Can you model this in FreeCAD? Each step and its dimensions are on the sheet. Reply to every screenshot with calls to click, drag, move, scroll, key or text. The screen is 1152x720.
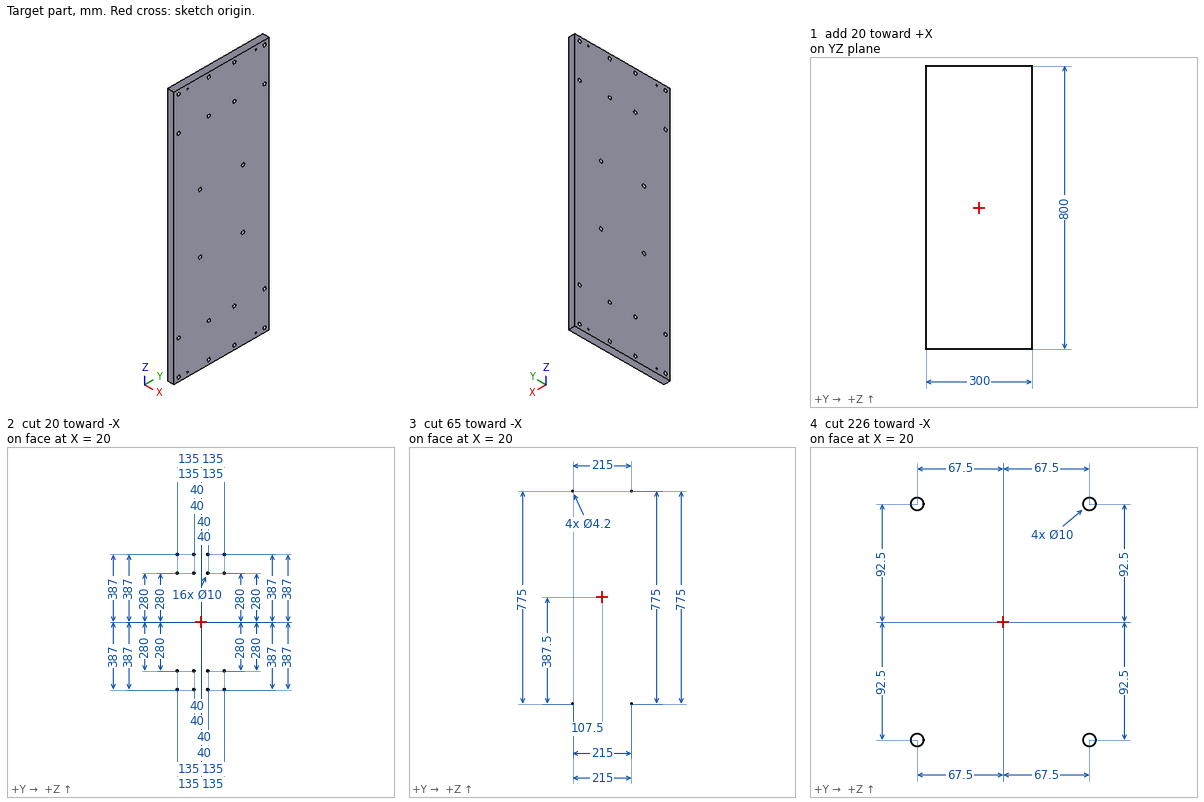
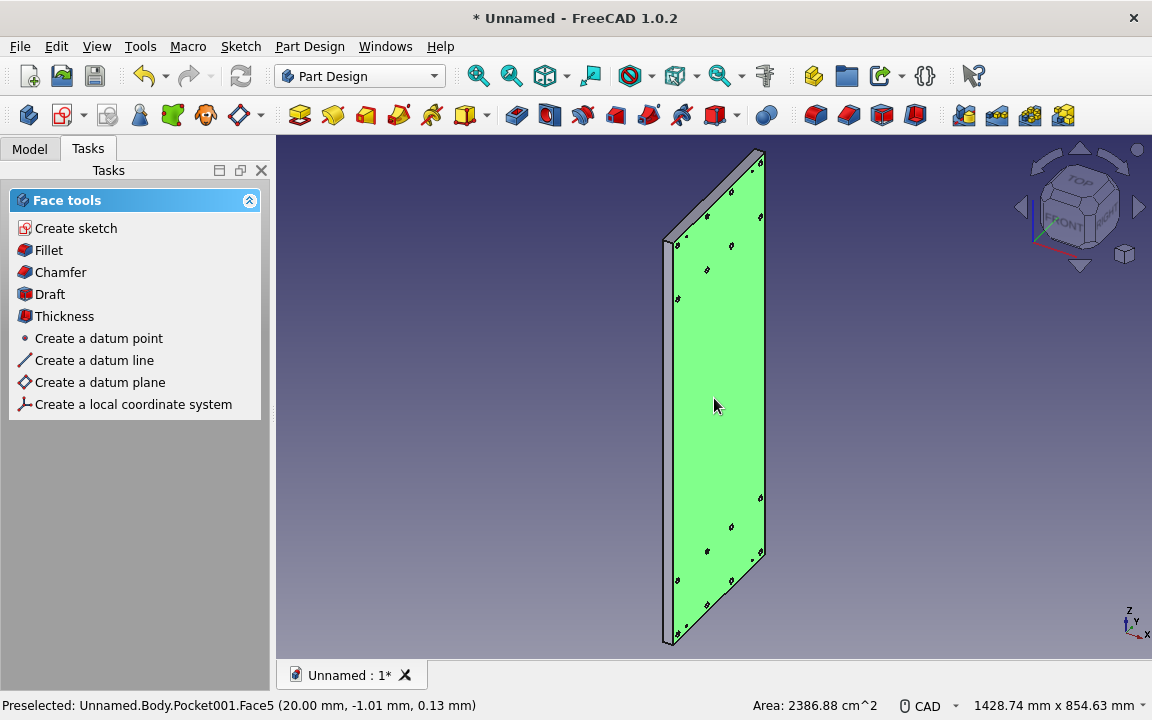
click(62, 116)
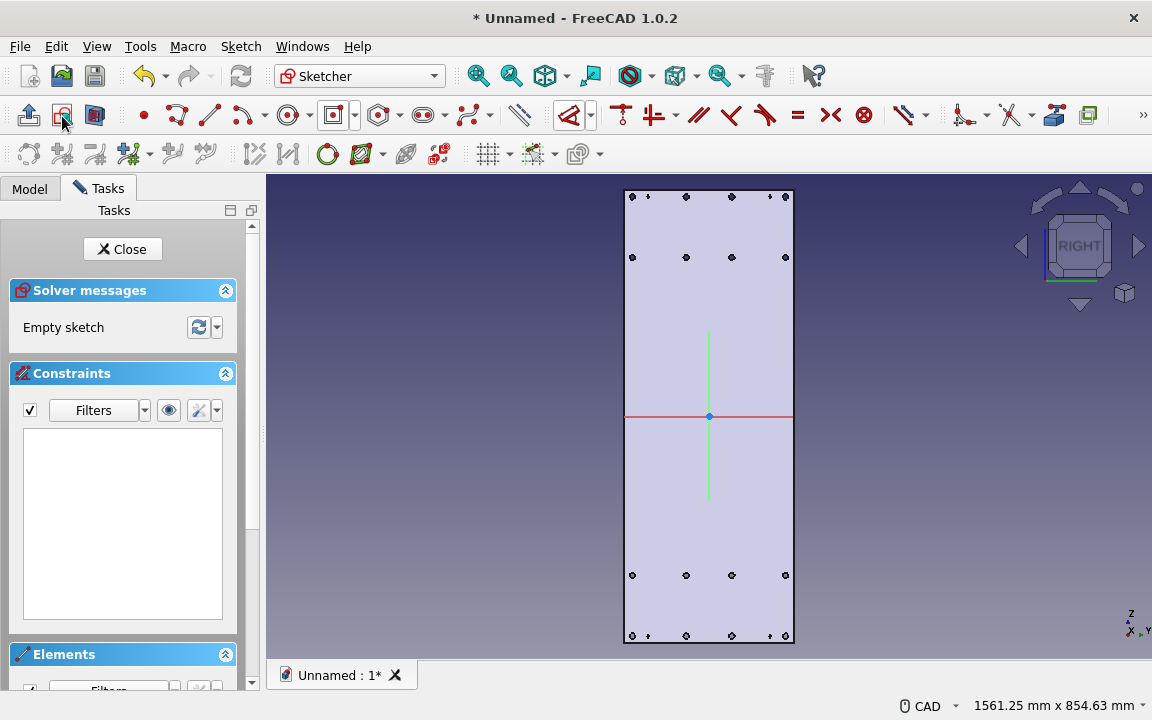
scroll(749, 416, up, 5)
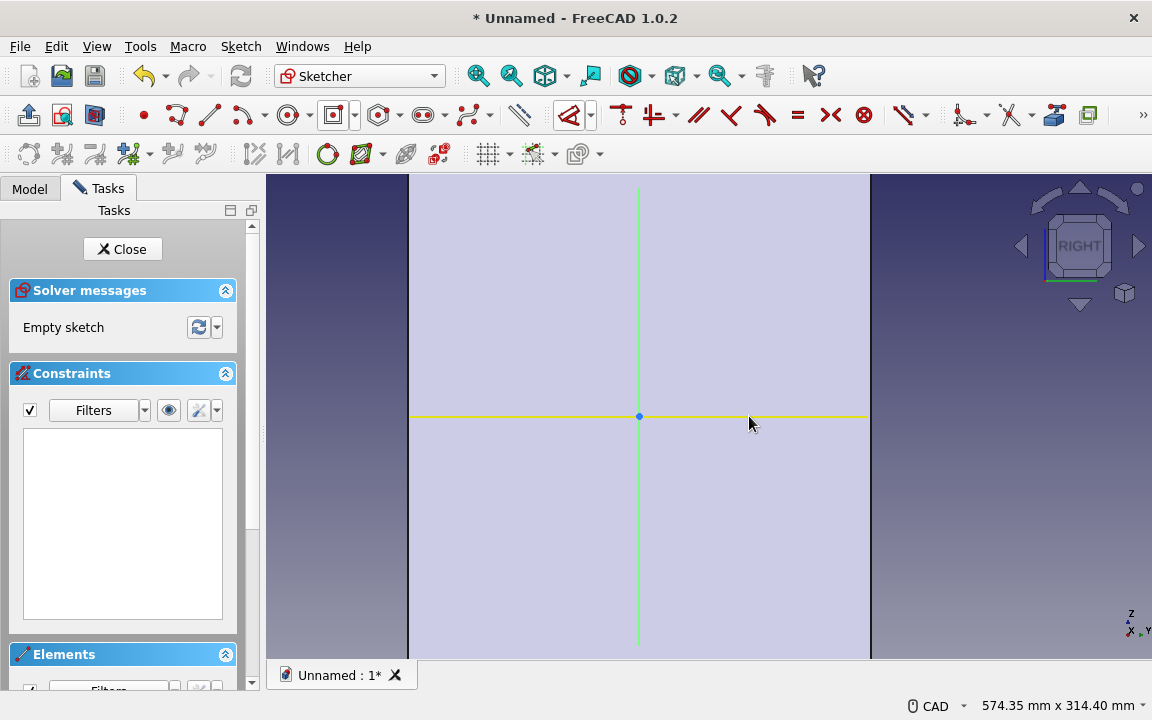
key(g)
key(c)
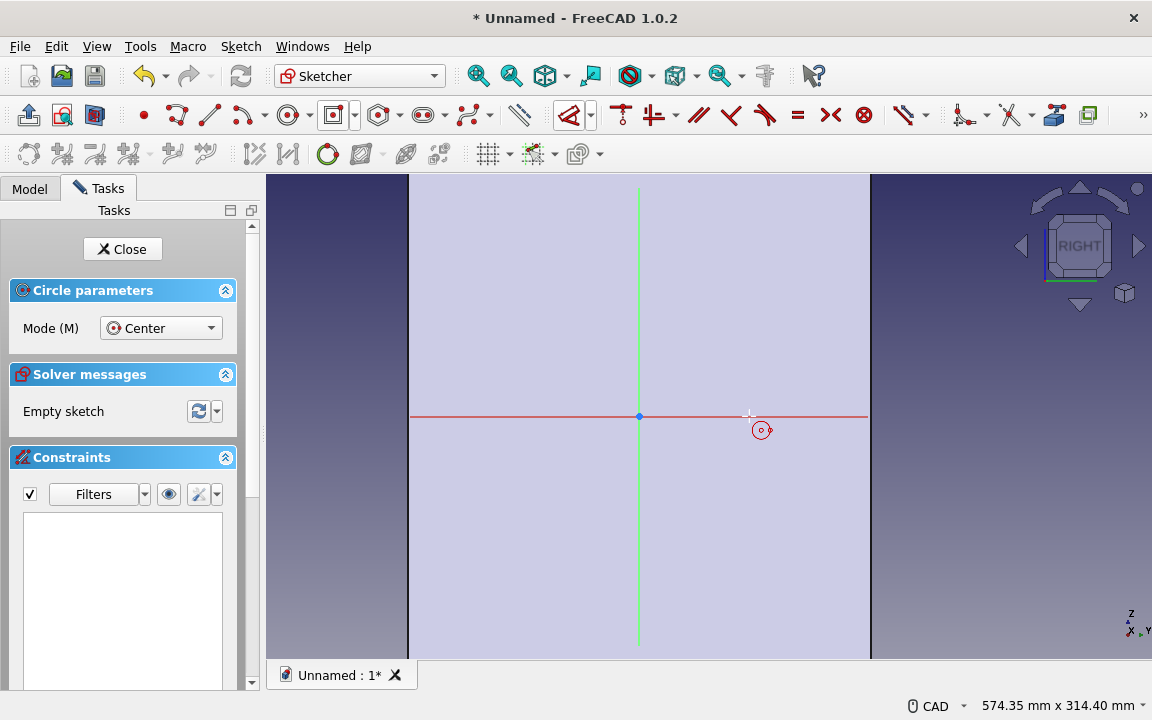
scroll(743, 274, up, 6)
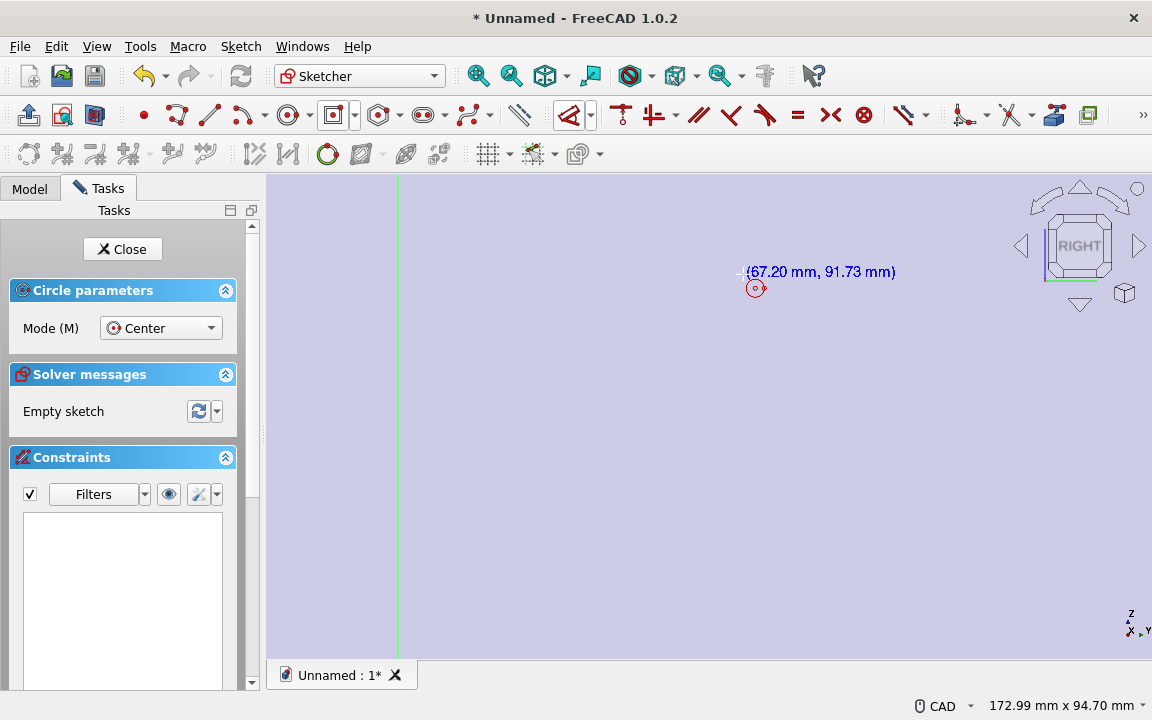
click(743, 273)
move(761, 255)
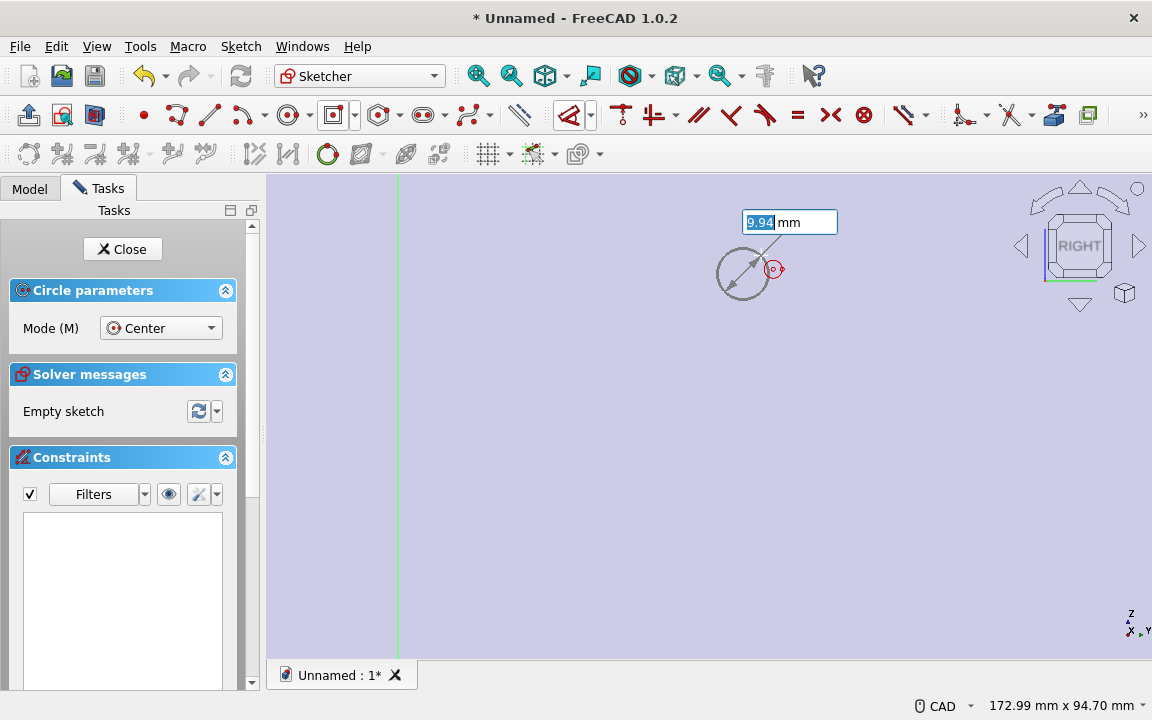
text(10)
key(Return)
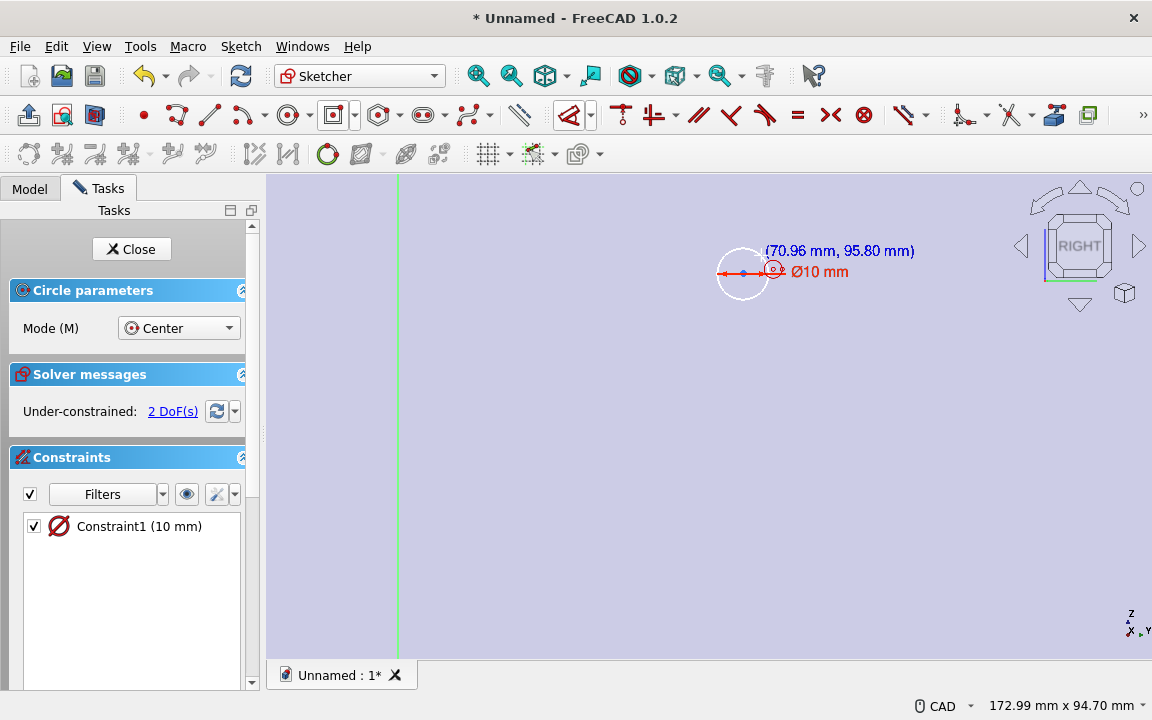
scroll(745, 274, down, 6)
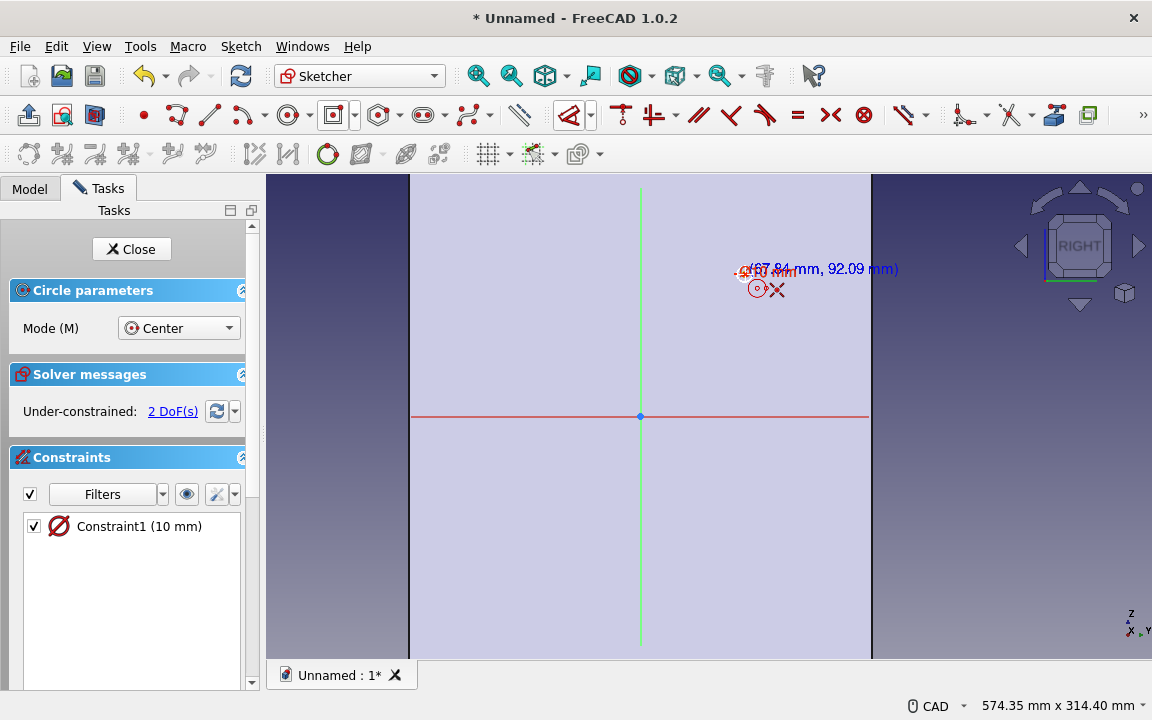
scroll(745, 559, up, 6)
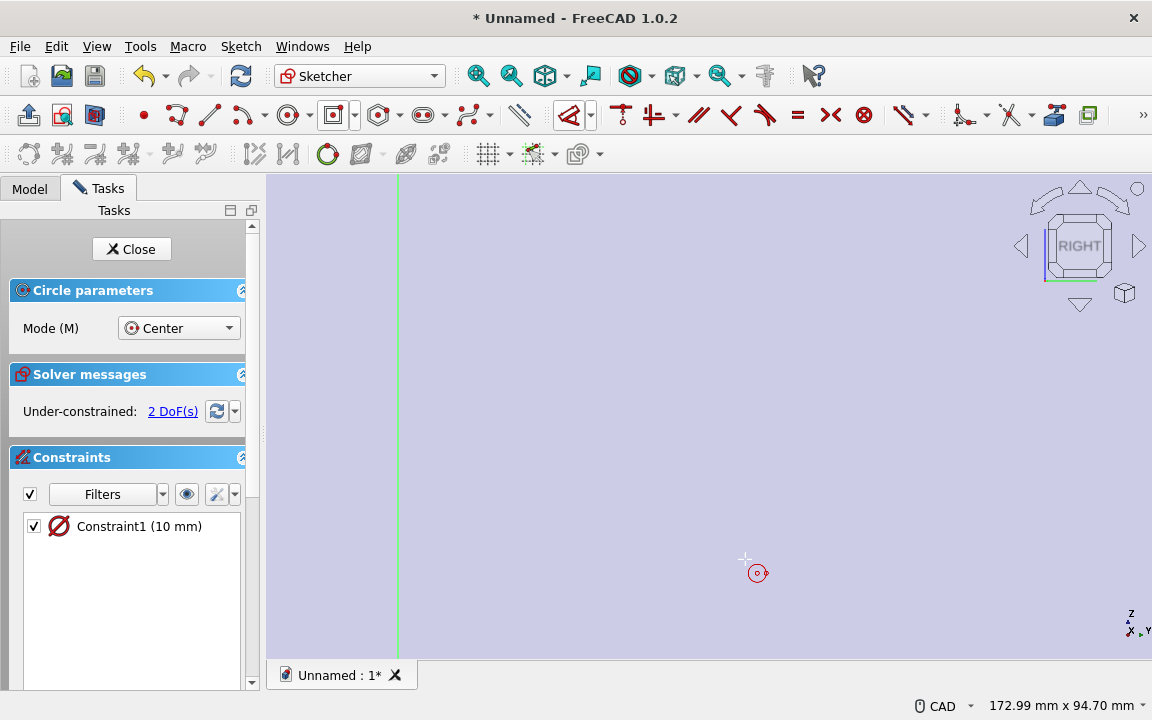
click(743, 558)
move(761, 540)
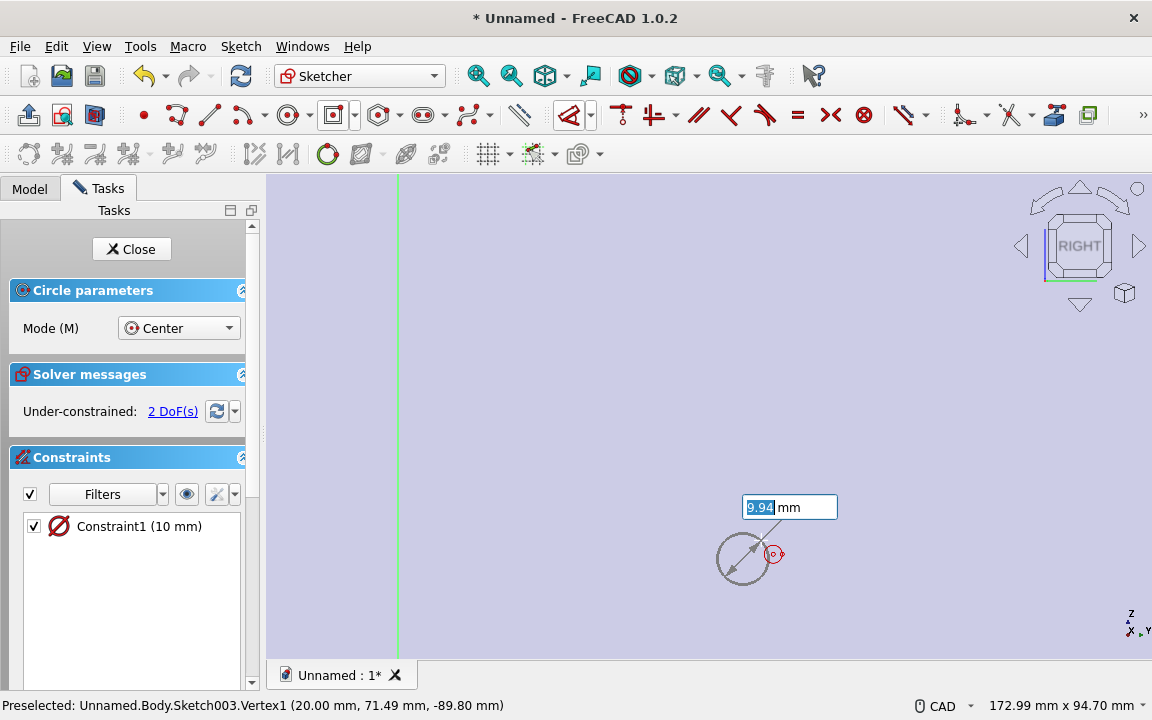
text(10)
key(Return)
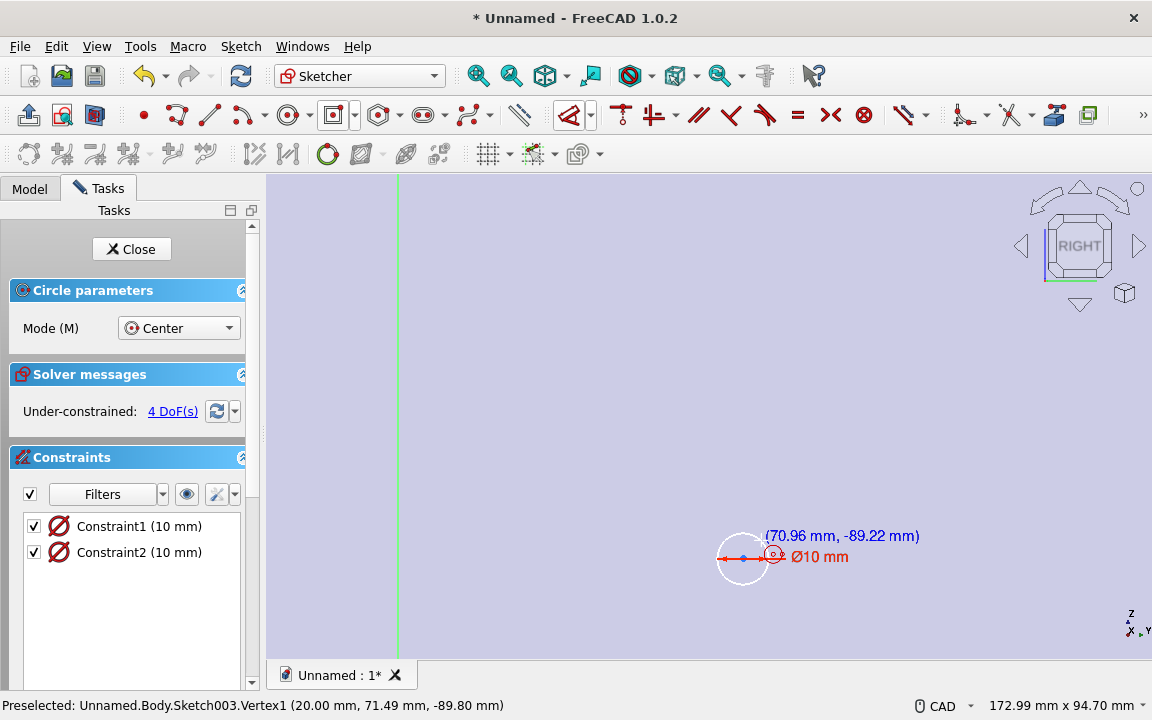
scroll(745, 560, down, 6)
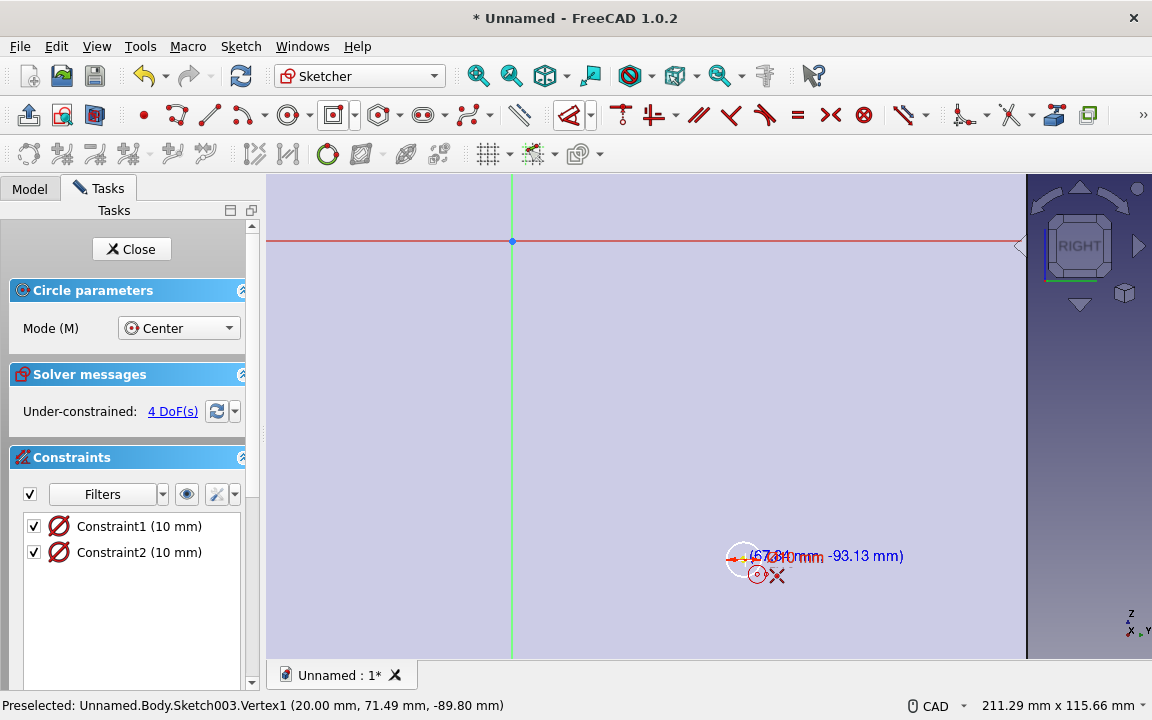
scroll(537, 560, up, 6)